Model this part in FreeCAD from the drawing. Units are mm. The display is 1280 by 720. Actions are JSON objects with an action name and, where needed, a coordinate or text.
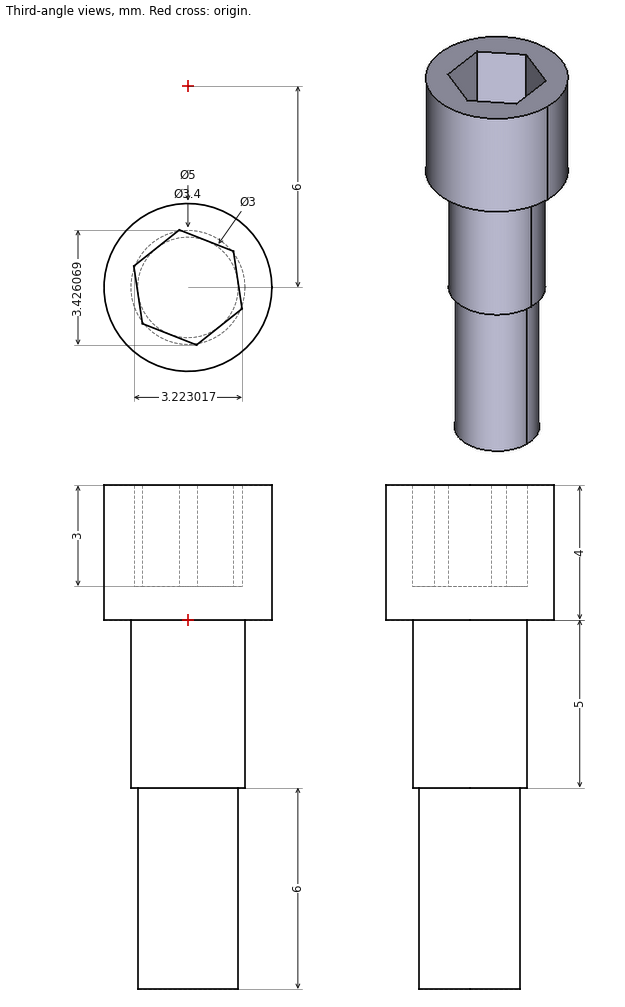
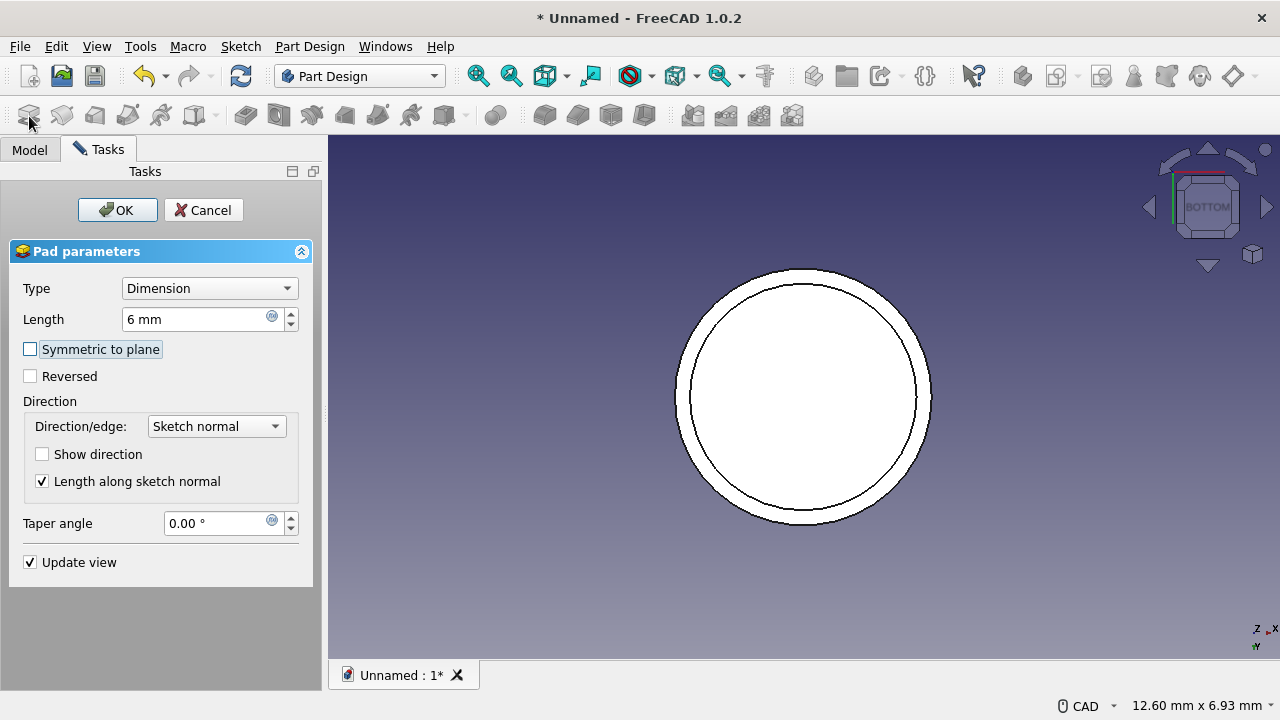
{"action": "left_click", "coordinate": [118, 210]}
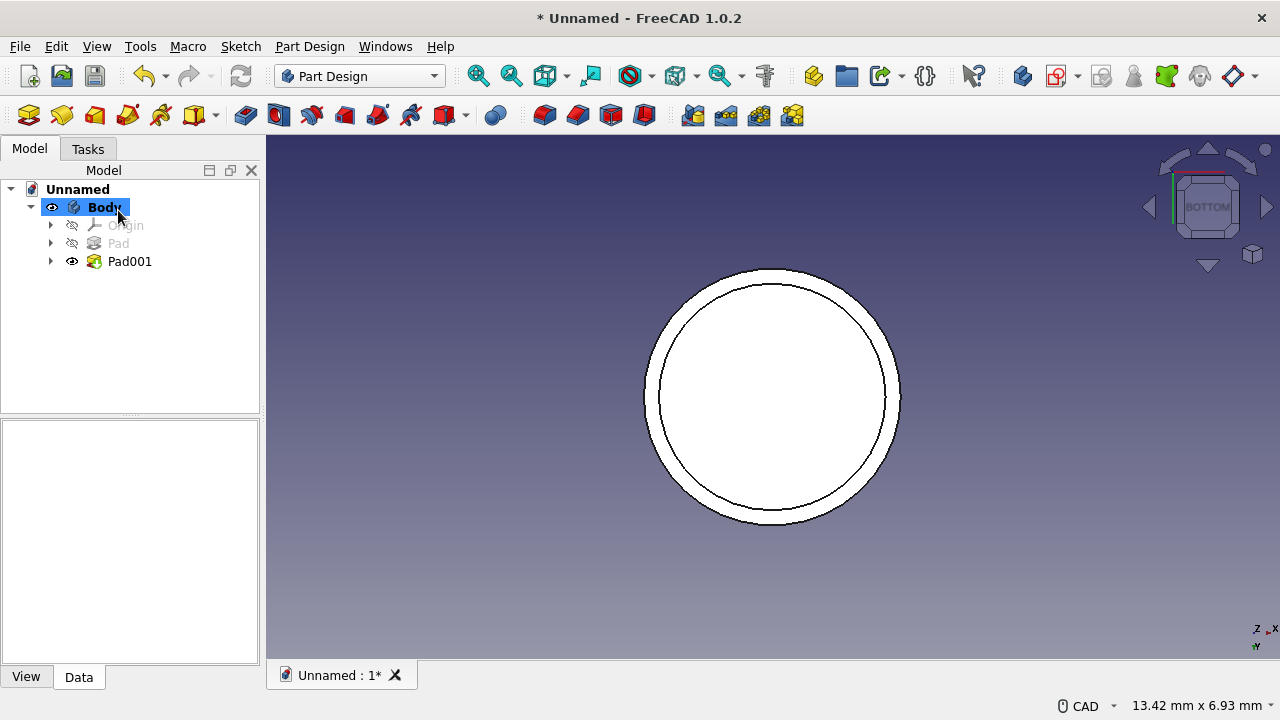
{"action": "left_click", "coordinate": [1056, 76]}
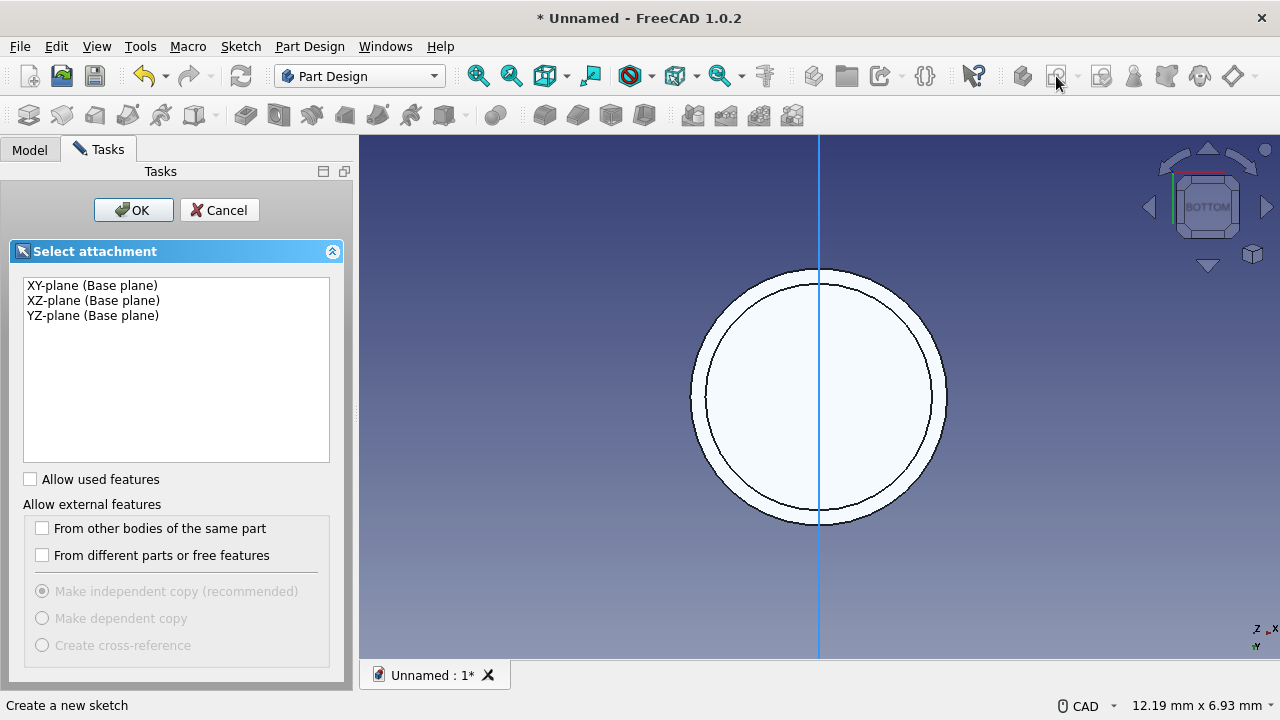
{"action": "left_click", "coordinate": [84, 286]}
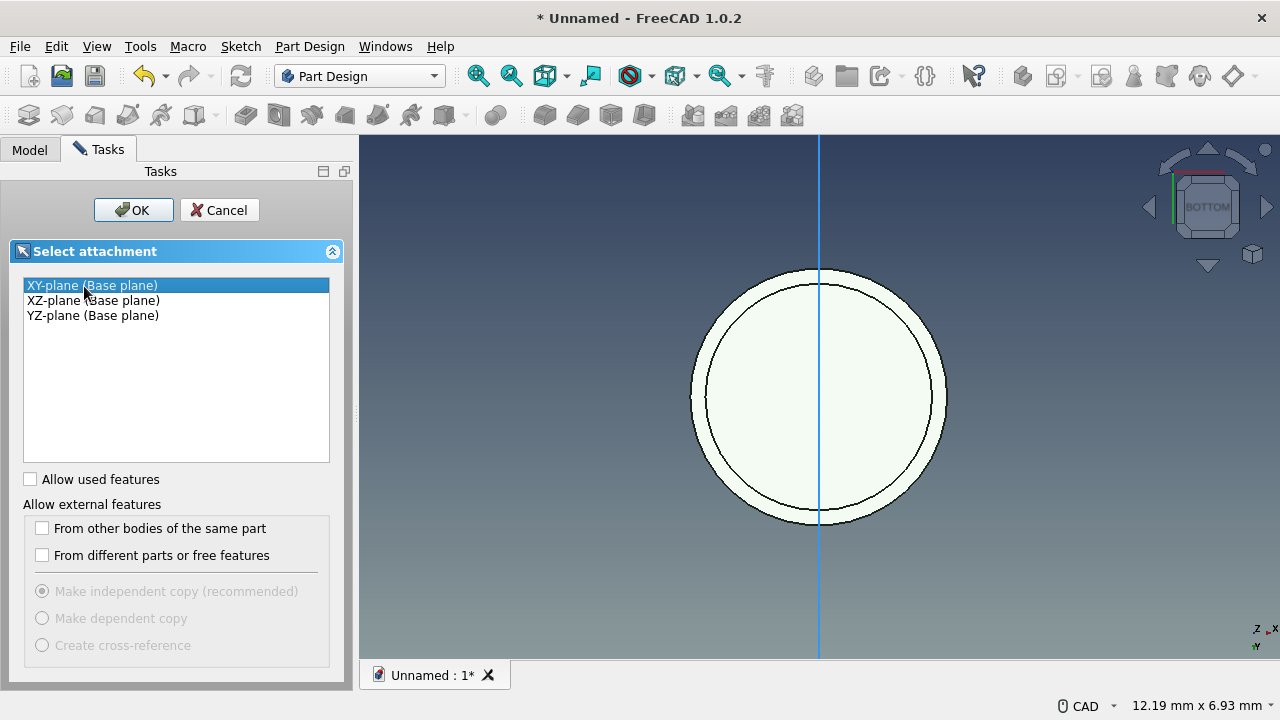
{"action": "left_click", "coordinate": [134, 210]}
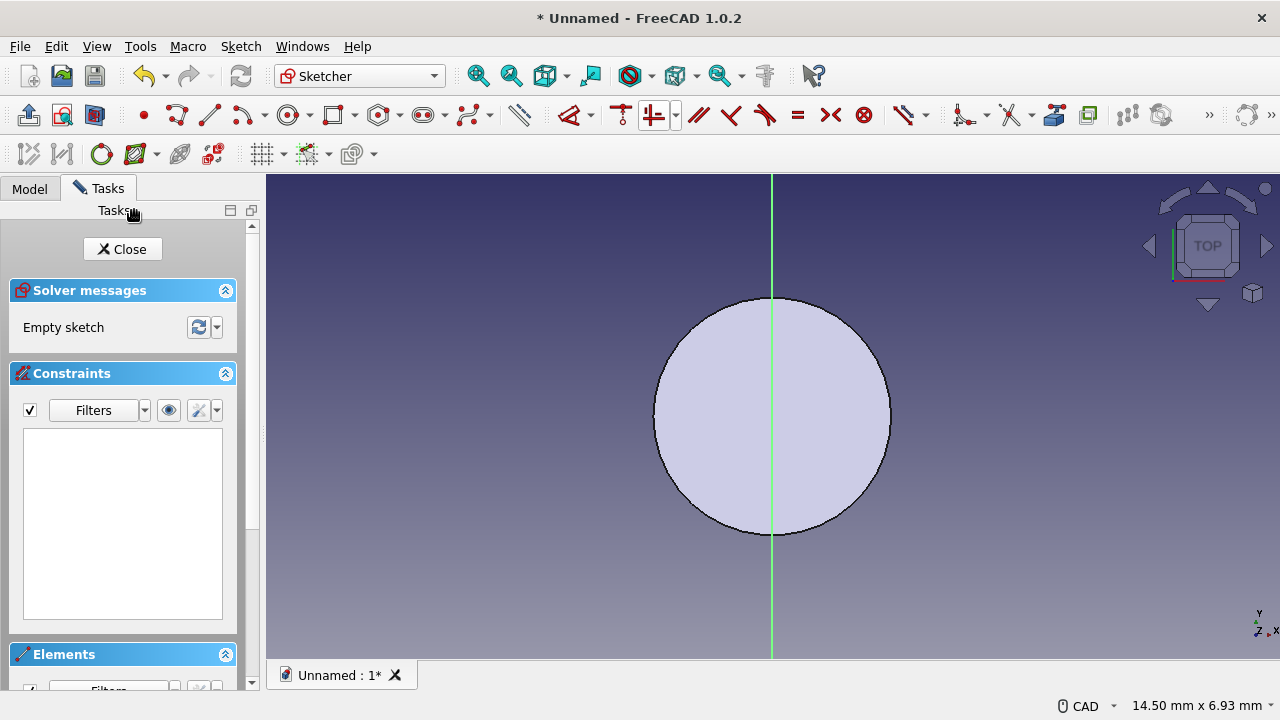
{"action": "scroll", "coordinate": [622, 565], "scroll_direction": "down", "scroll_amount": 3}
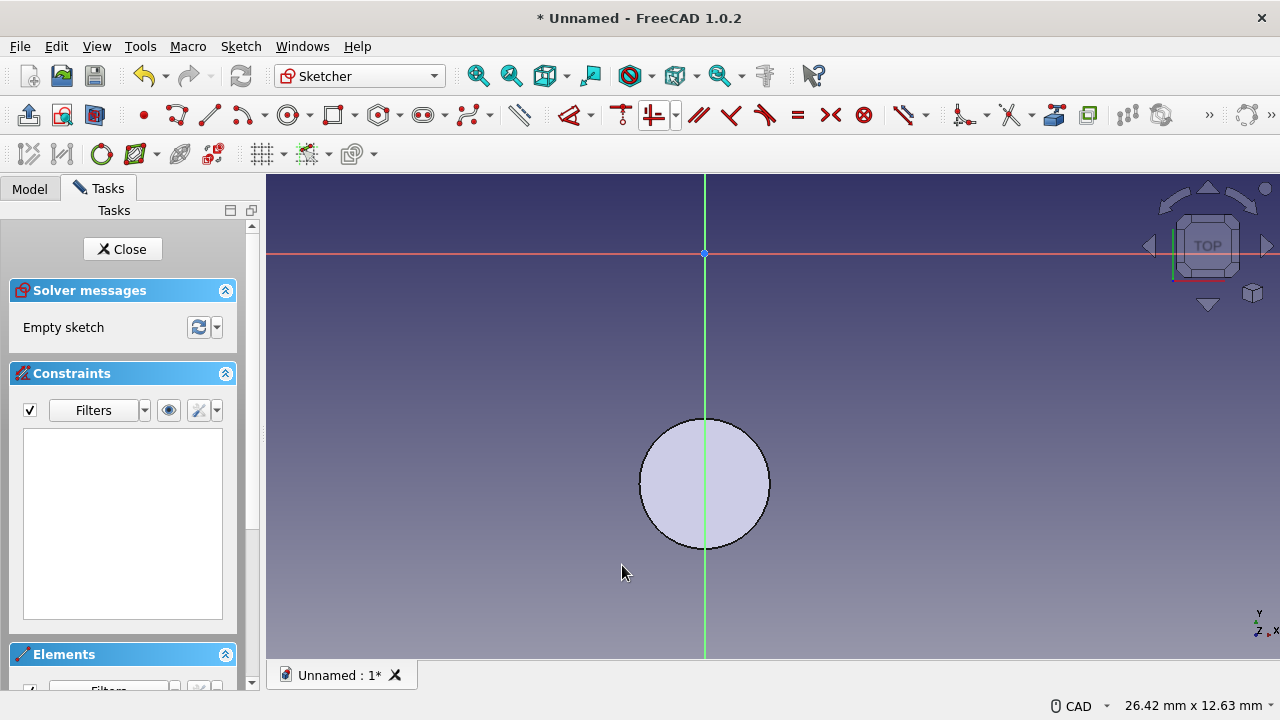
{"action": "key", "text": "g c"}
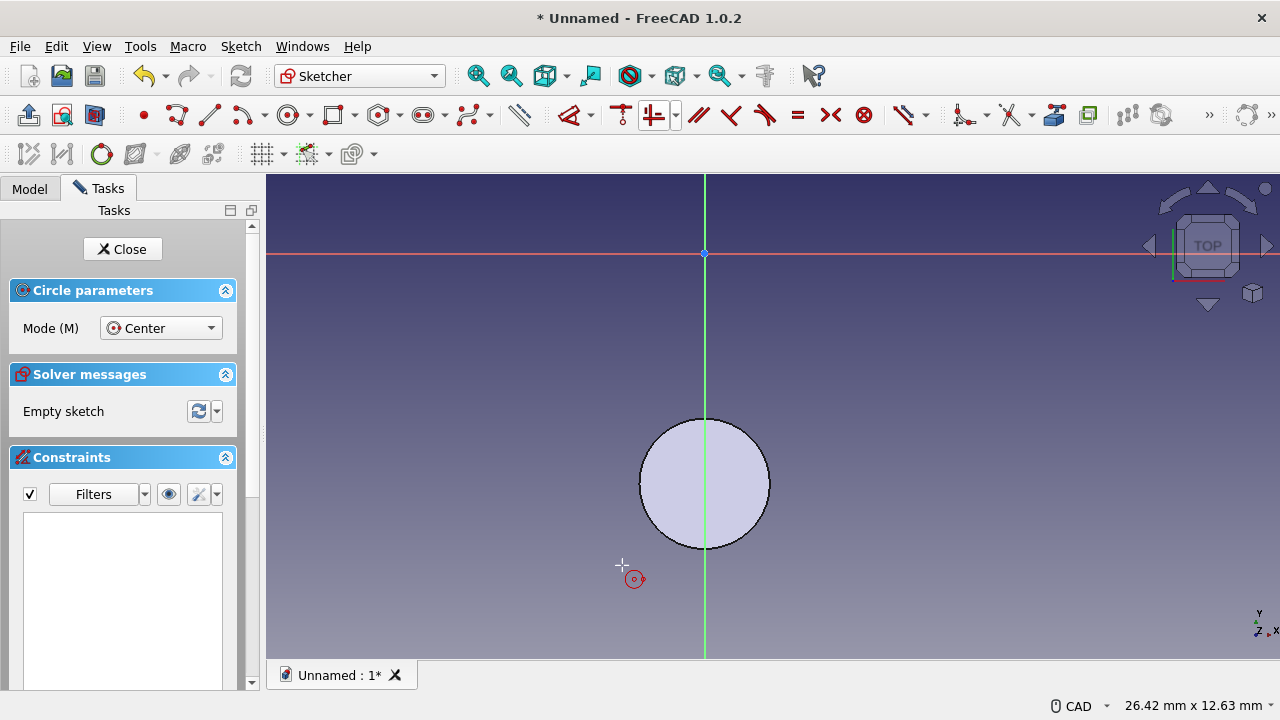
{"action": "left_click", "coordinate": [705, 484]}
{"action": "left_click", "coordinate": [773, 416]}
{"action": "key", "text": "Escape"}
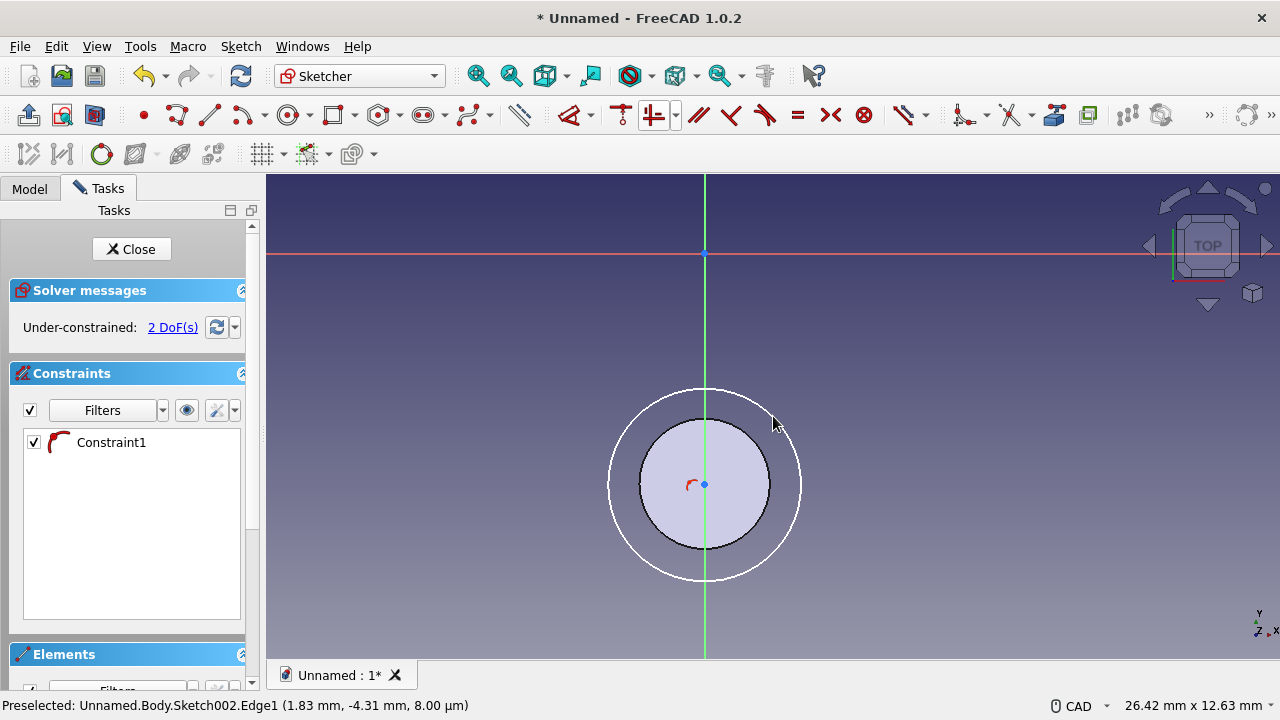
{"action": "key", "text": "d"}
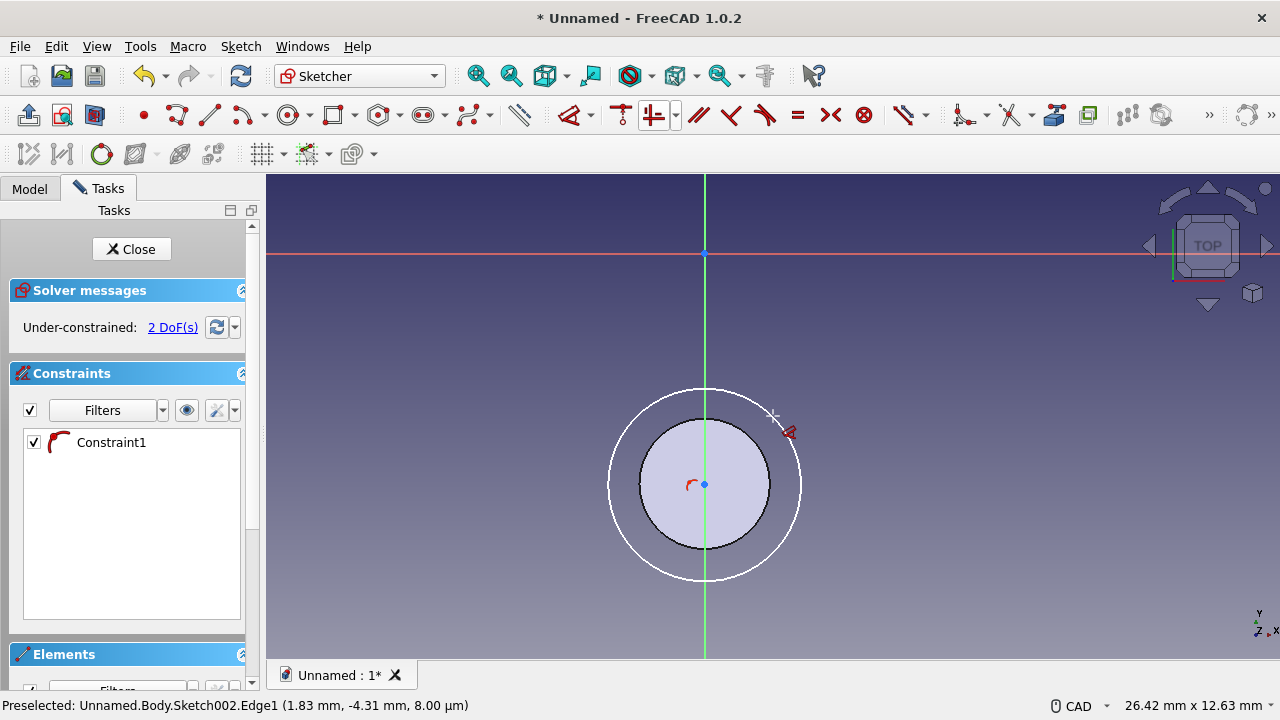
{"action": "left_click", "coordinate": [773, 417]}
{"action": "left_click", "coordinate": [796, 394]}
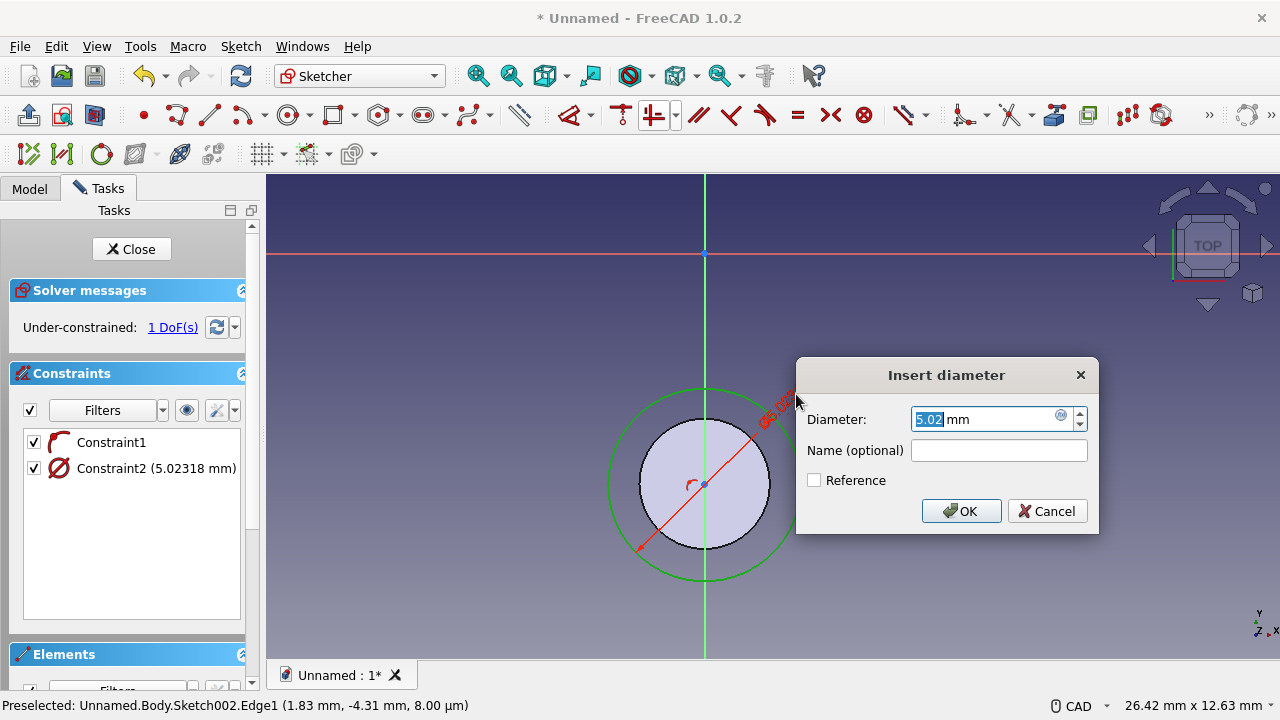
{"action": "type", "text": "5"}
{"action": "key", "text": "Return"}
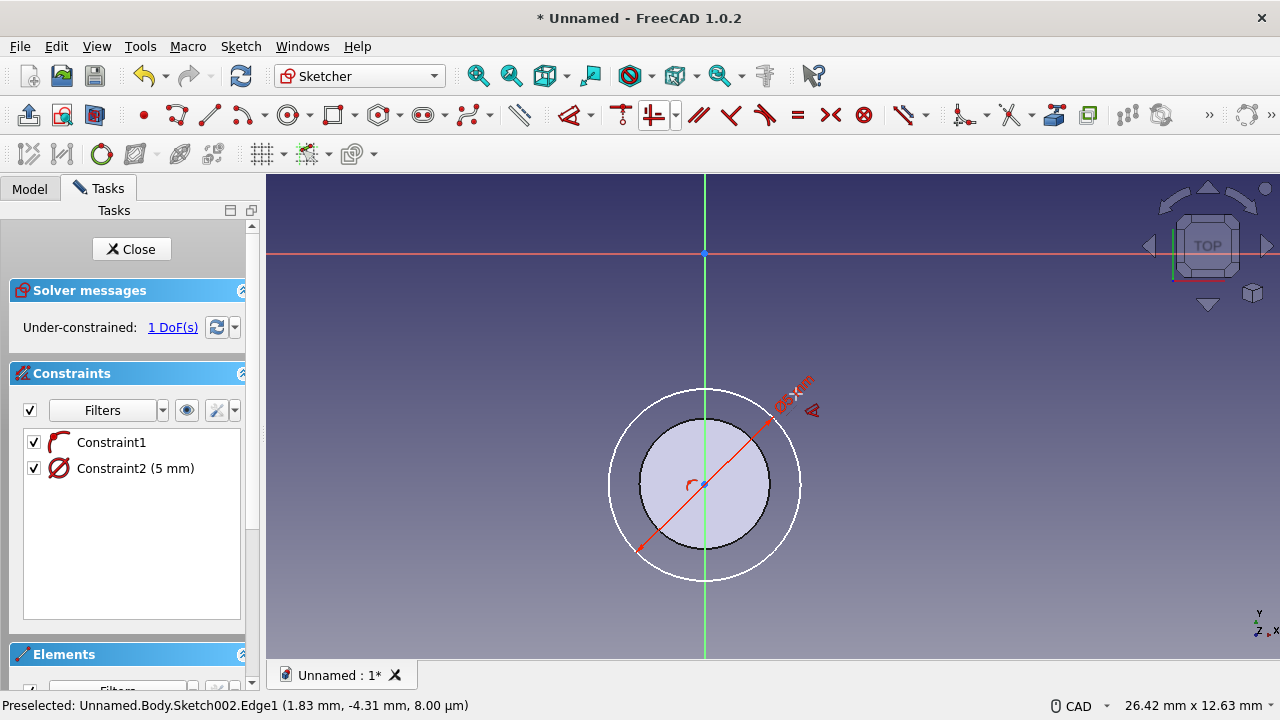
{"action": "left_click", "coordinate": [705, 485]}
{"action": "left_click", "coordinate": [739, 369]}